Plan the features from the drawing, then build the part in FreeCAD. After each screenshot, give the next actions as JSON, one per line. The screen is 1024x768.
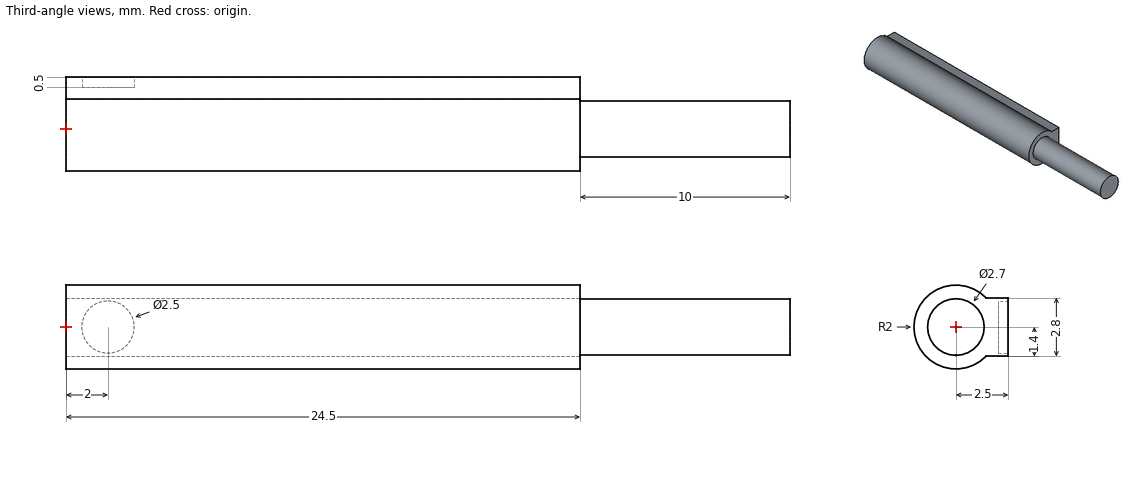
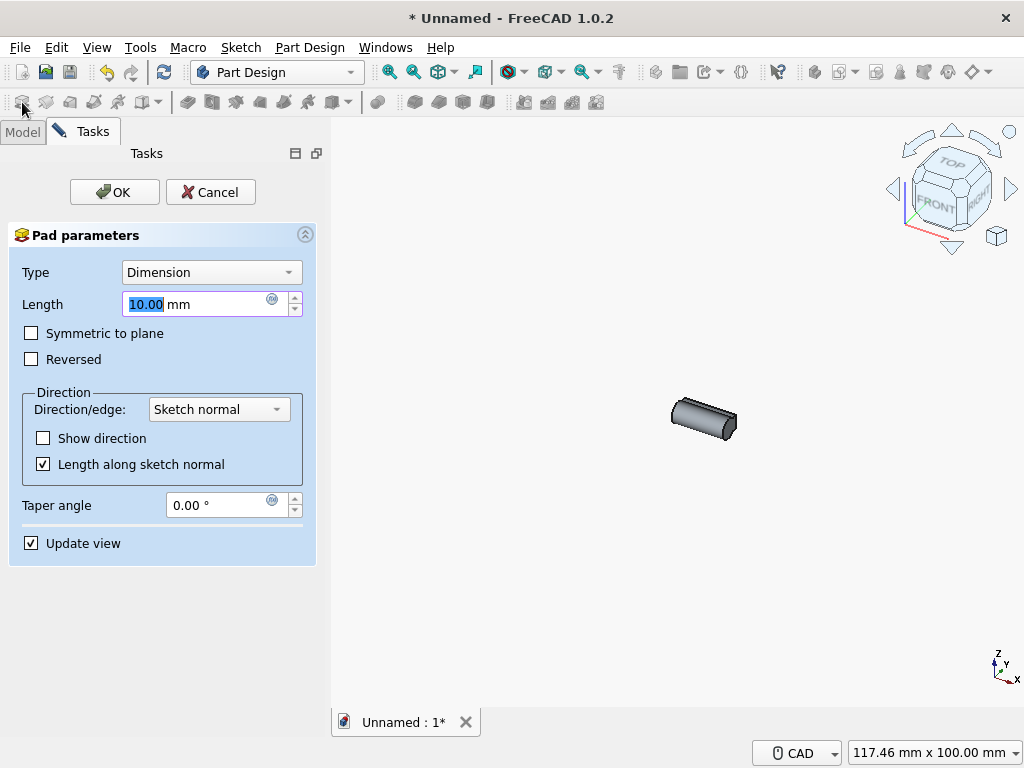
{"action": "type", "text": "24.5"}
{"action": "key", "text": "Tab"}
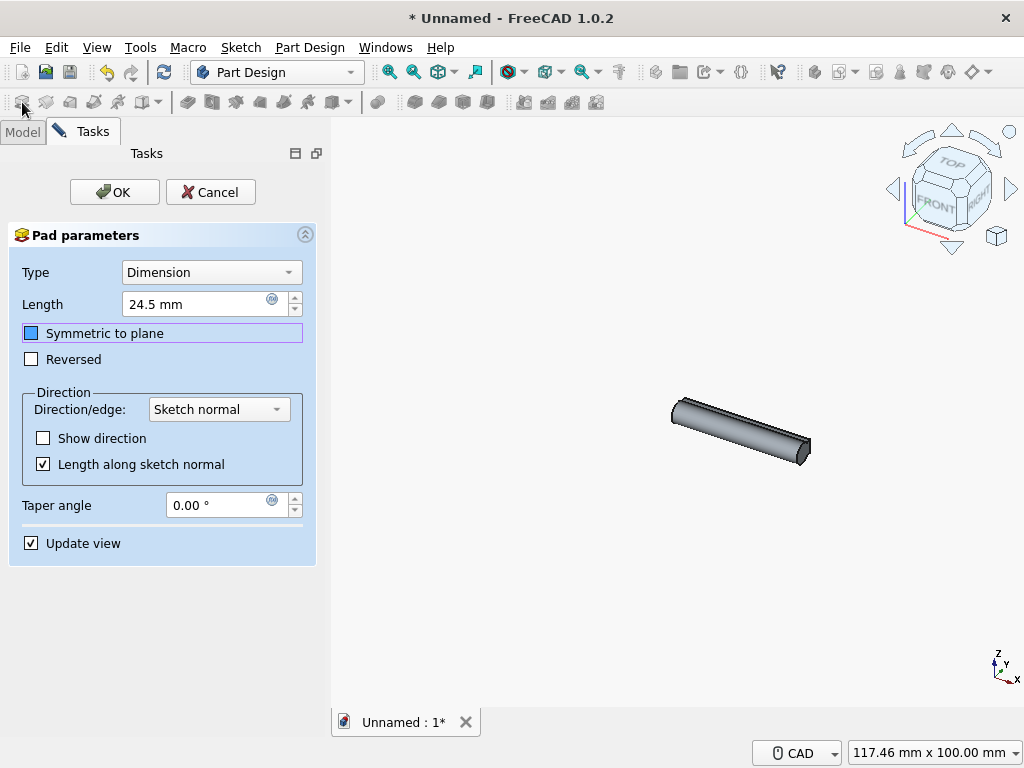
{"action": "left_click", "coordinate": [115, 192]}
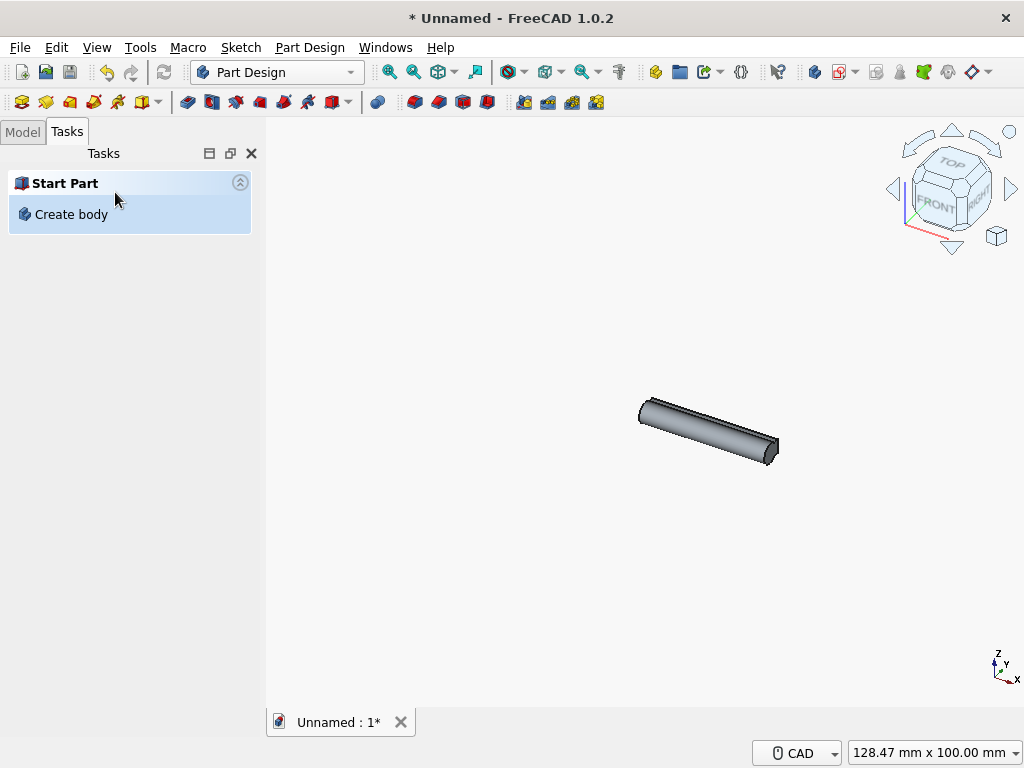
{"action": "key", "text": "v f"}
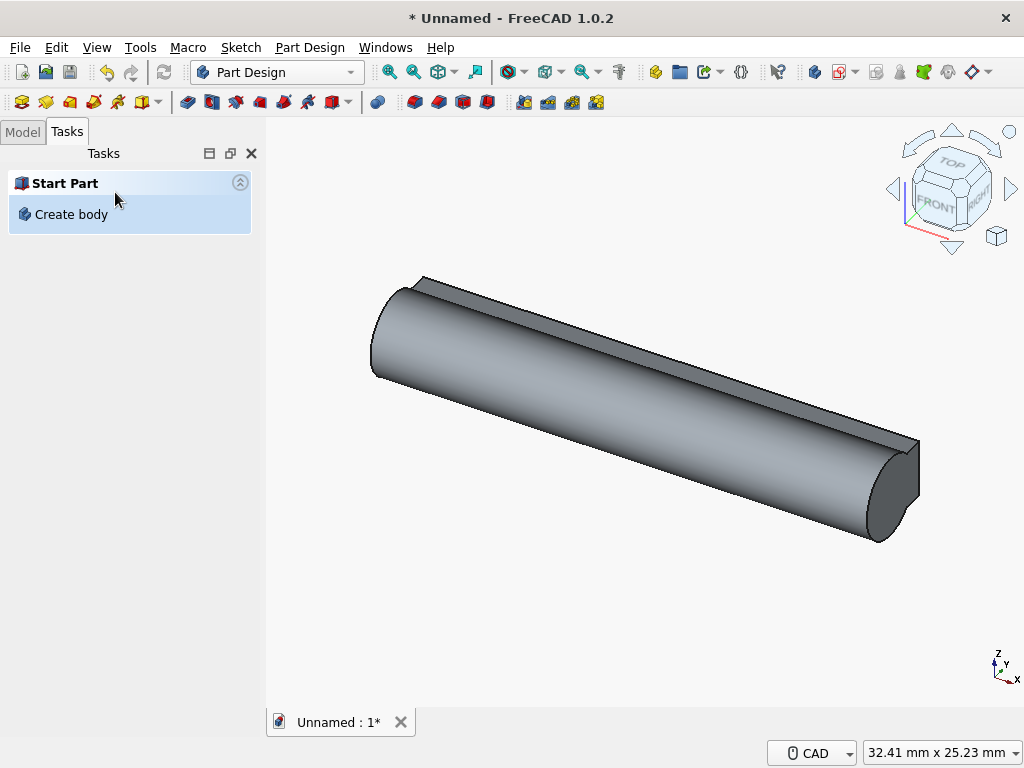
{"action": "left_click", "coordinate": [893, 493]}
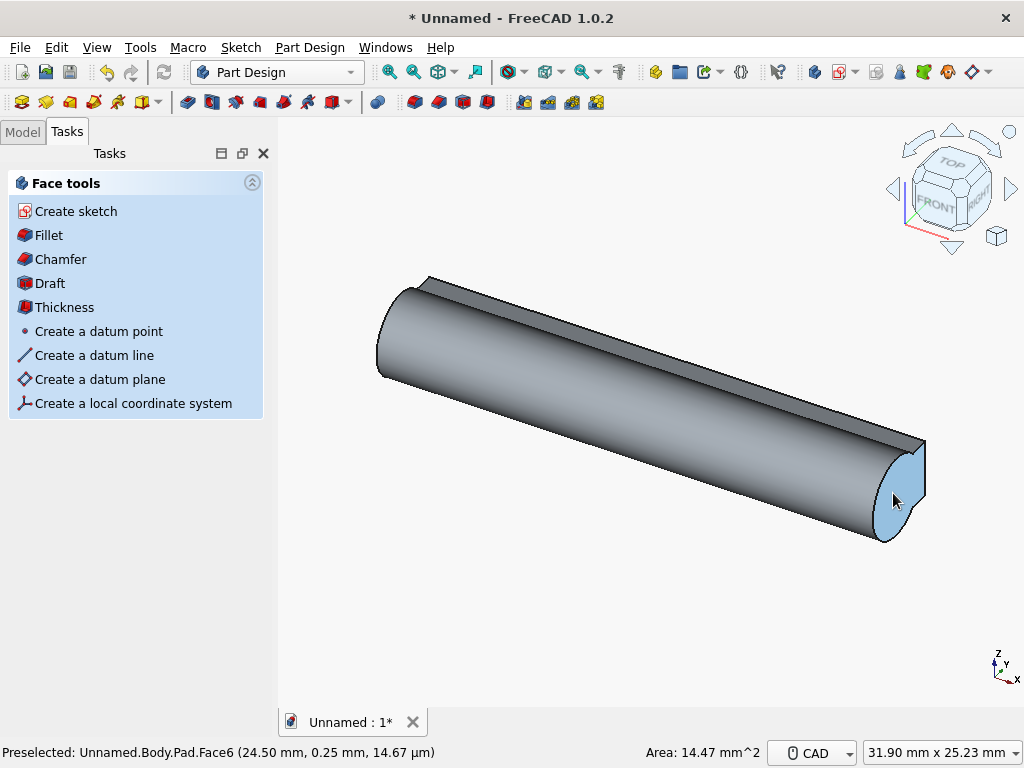
{"action": "left_click", "coordinate": [840, 72]}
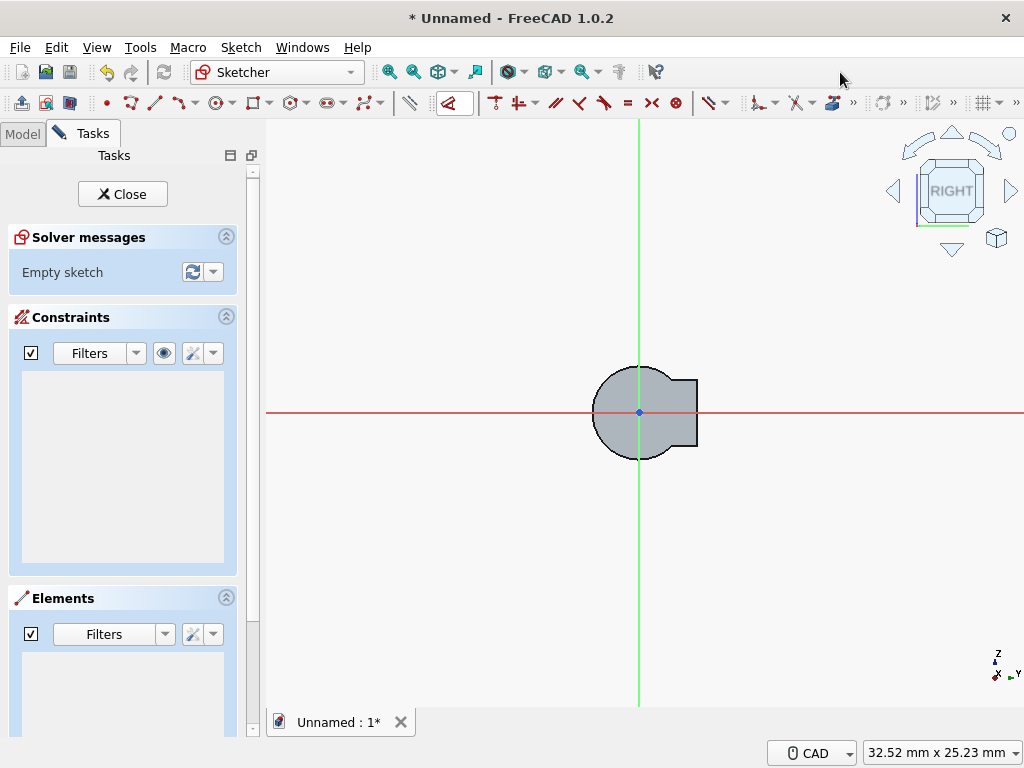
{"action": "scroll", "coordinate": [651, 413], "scroll_direction": "up", "scroll_amount": 9}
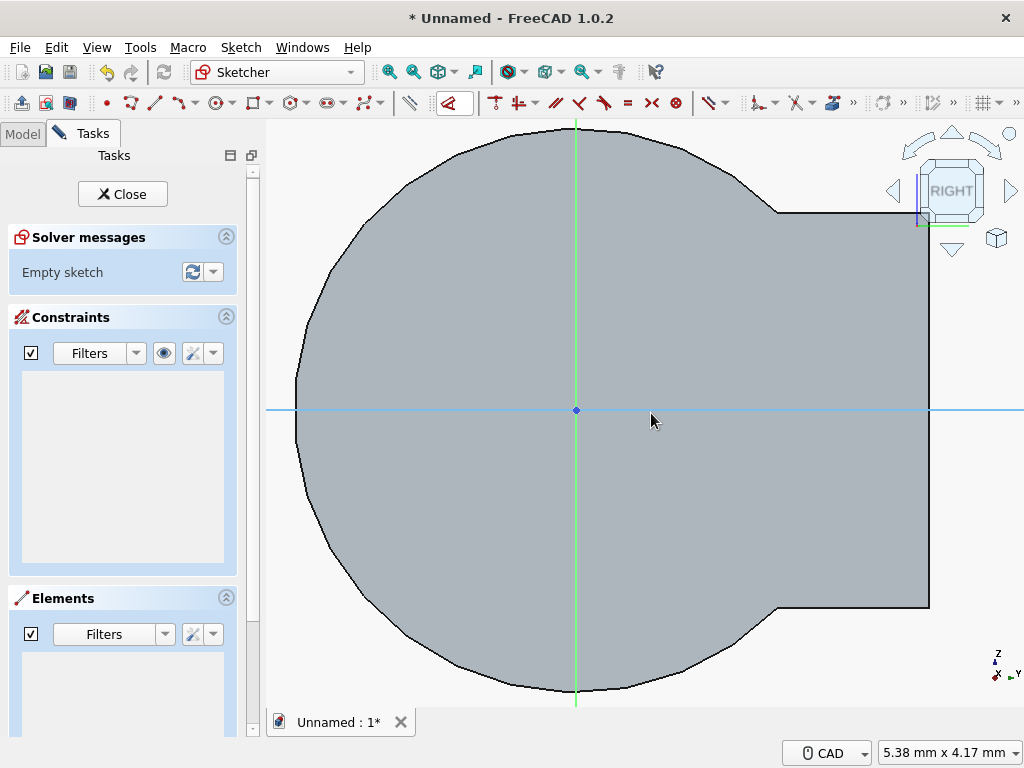
{"action": "left_click", "coordinate": [216, 104]}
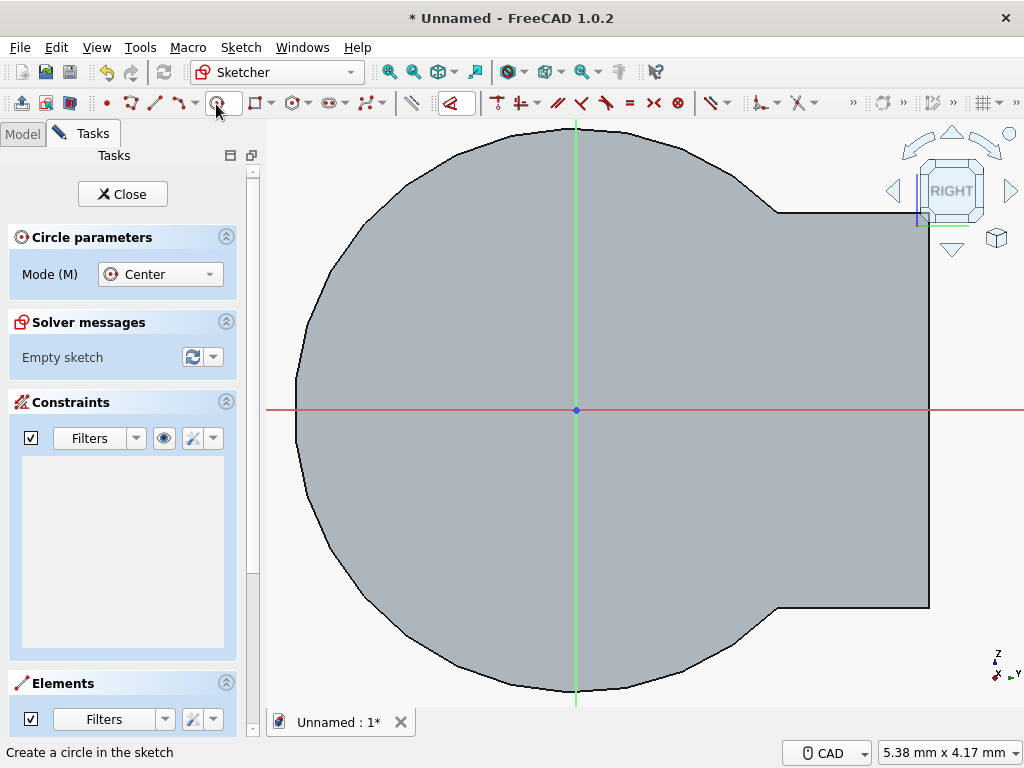
{"action": "left_click", "coordinate": [576, 410]}
{"action": "mouse_move", "coordinate": [711, 276]}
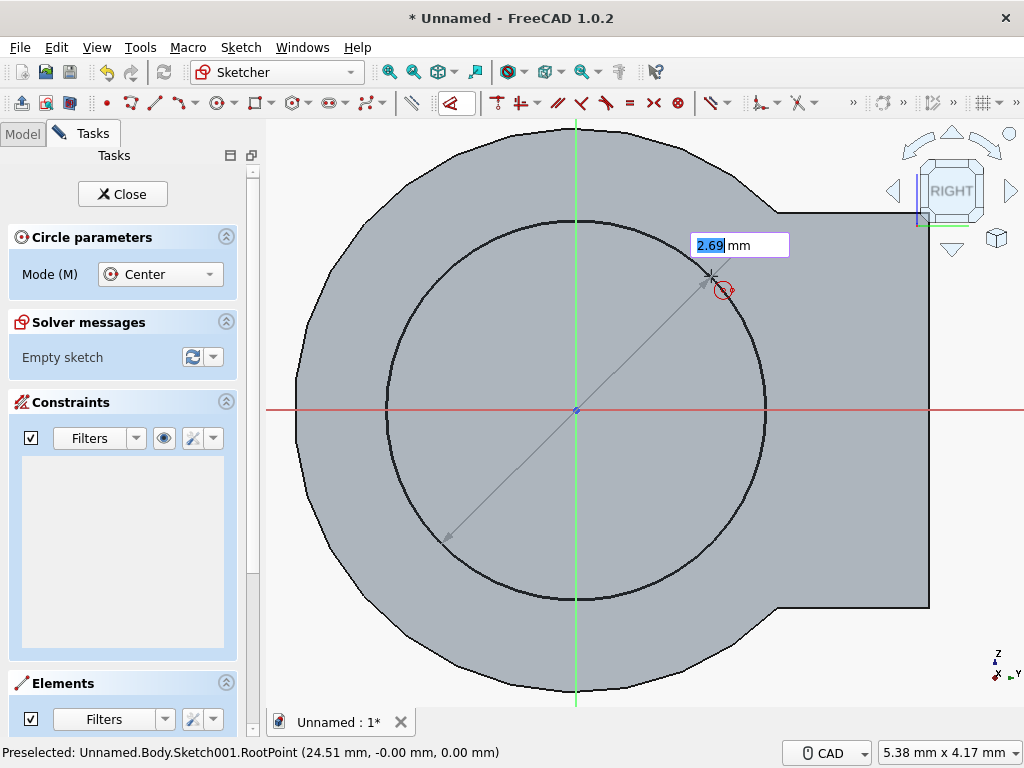
{"action": "type", "text": "2.7"}
{"action": "key", "text": "Return"}
{"action": "key", "text": "Escape"}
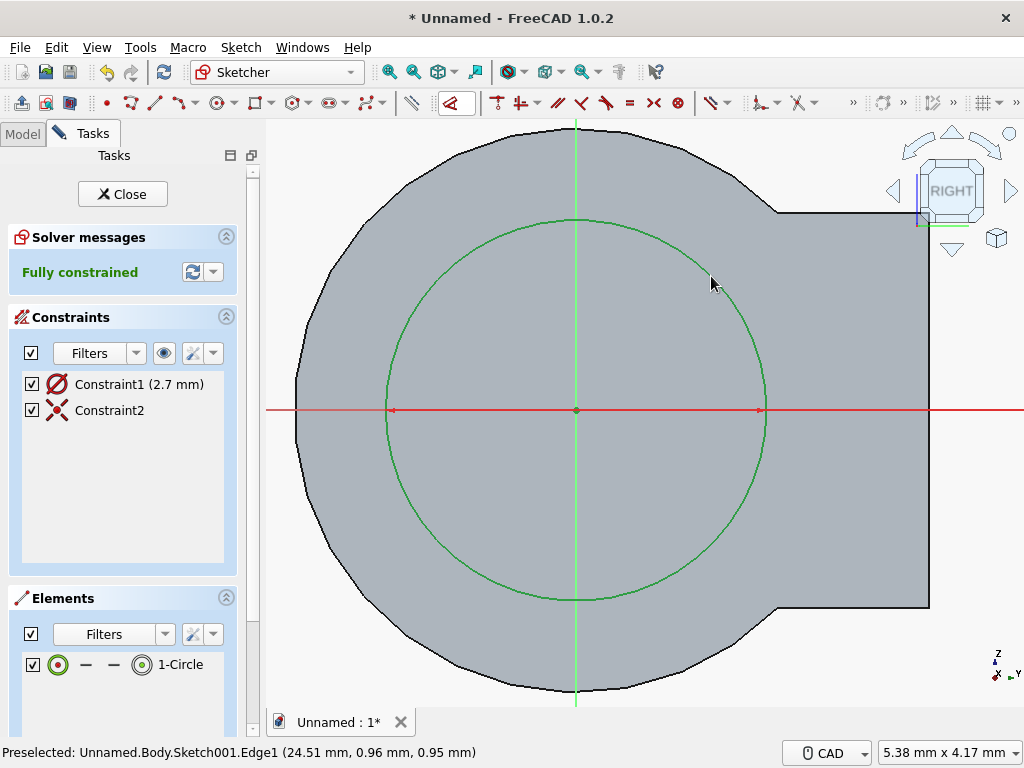
{"action": "left_click", "coordinate": [123, 194]}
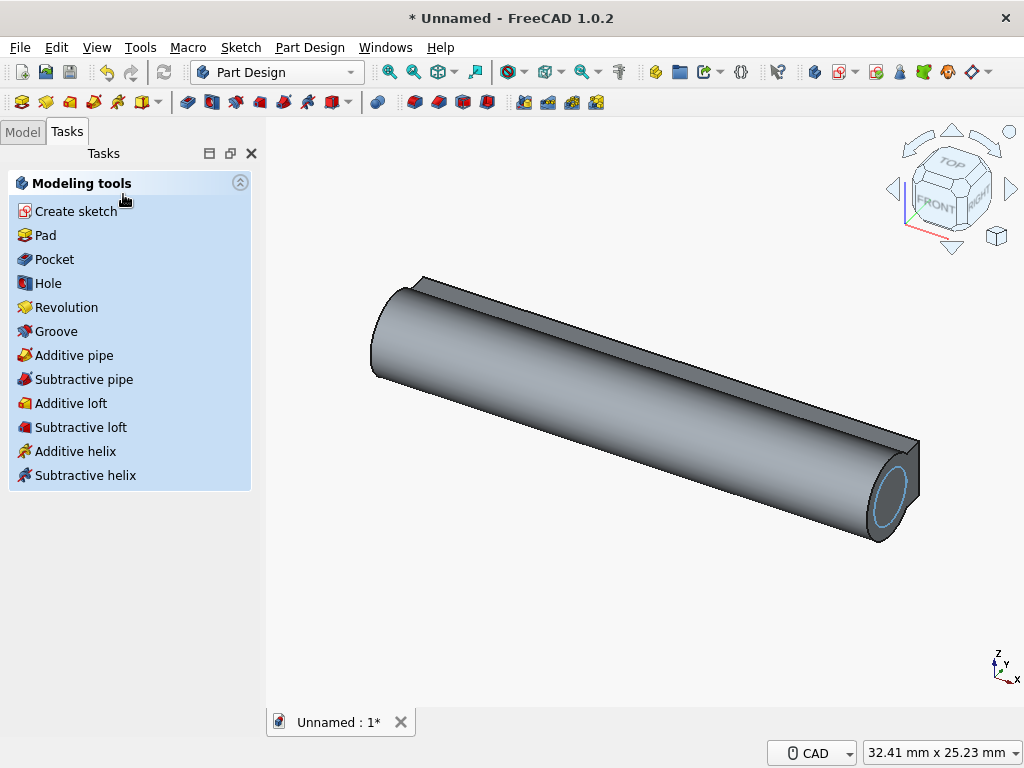
{"action": "left_click", "coordinate": [22, 102]}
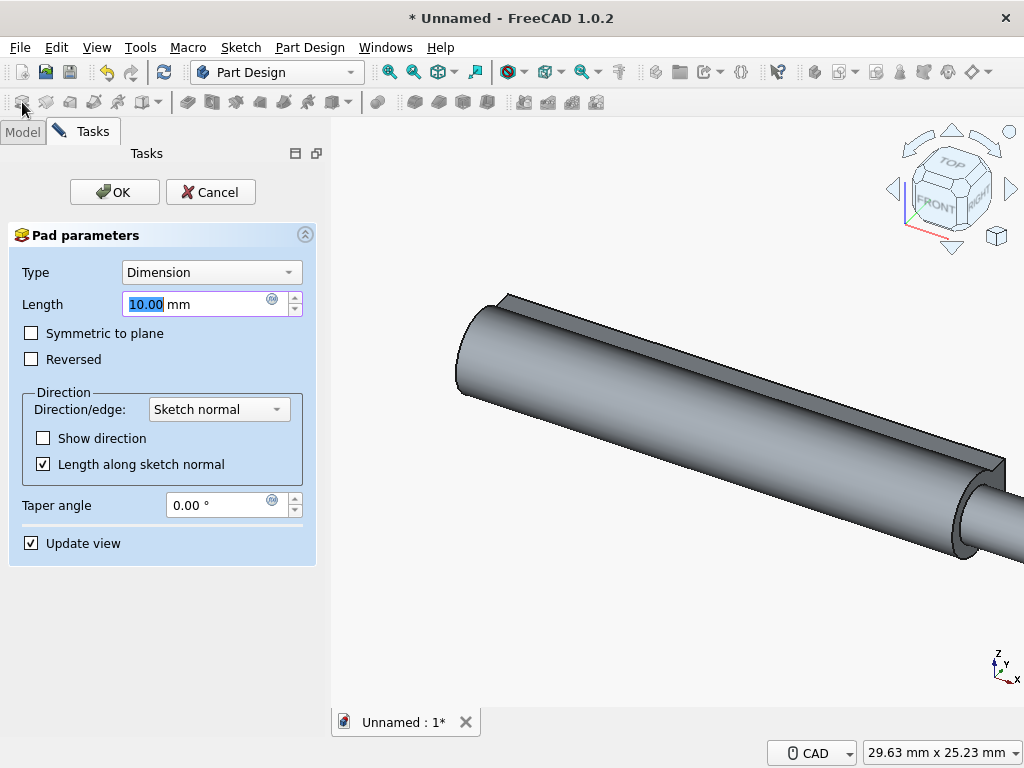
{"action": "type", "text": "10"}
{"action": "key", "text": "Tab"}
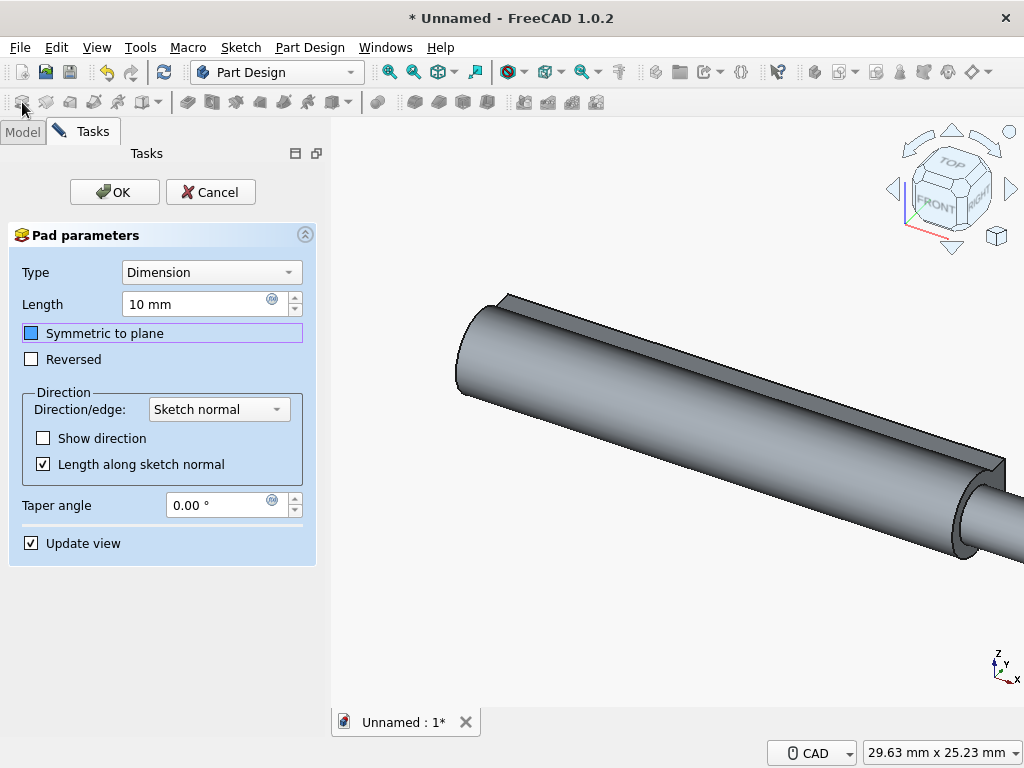
{"action": "left_click", "coordinate": [115, 192]}